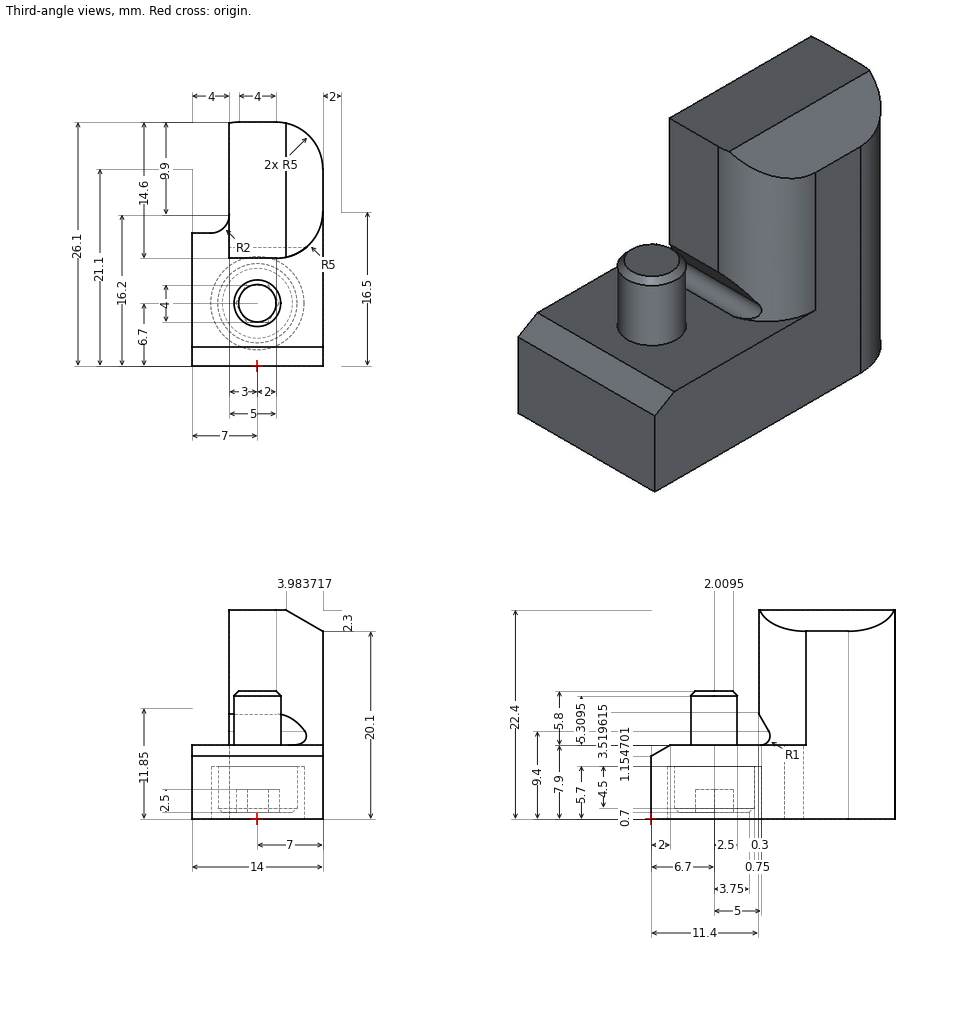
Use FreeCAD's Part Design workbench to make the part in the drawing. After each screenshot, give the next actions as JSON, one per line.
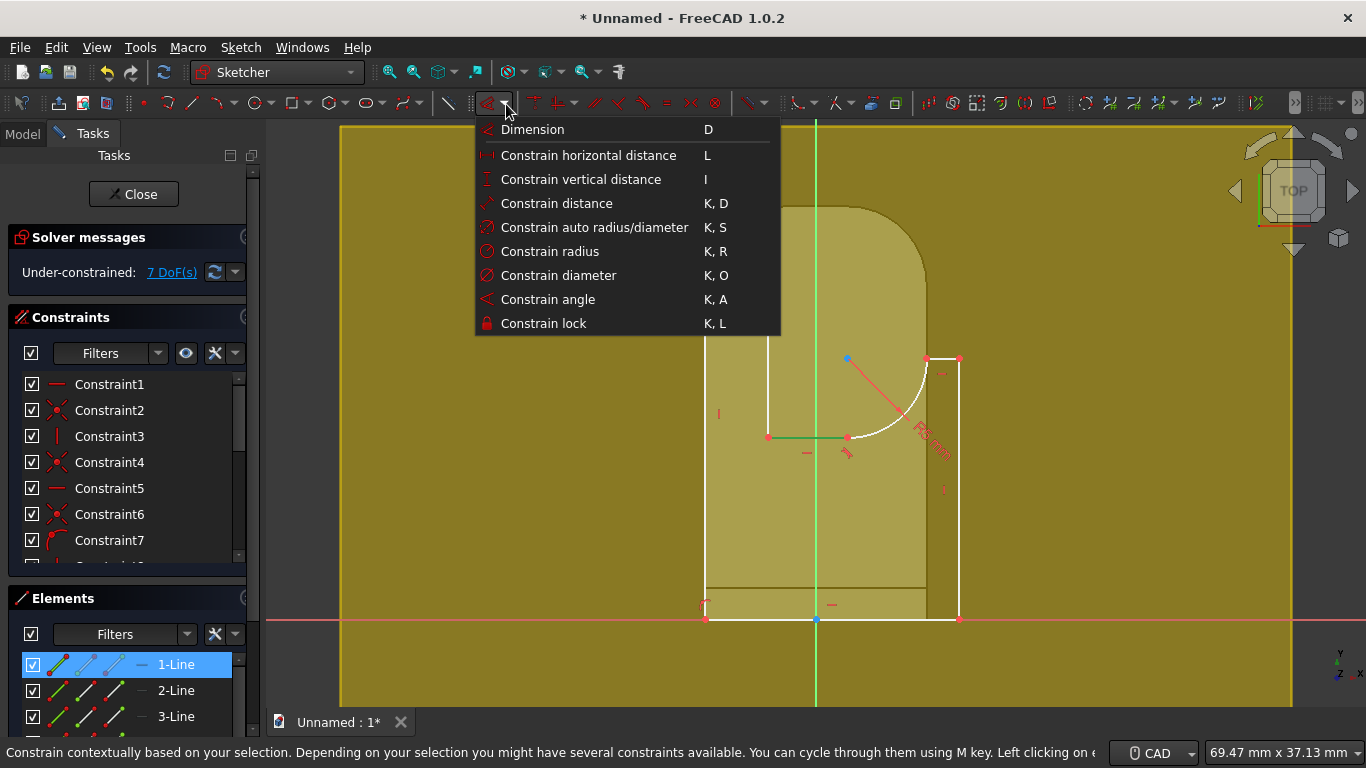
{"action": "left_click", "coordinate": [628, 155]}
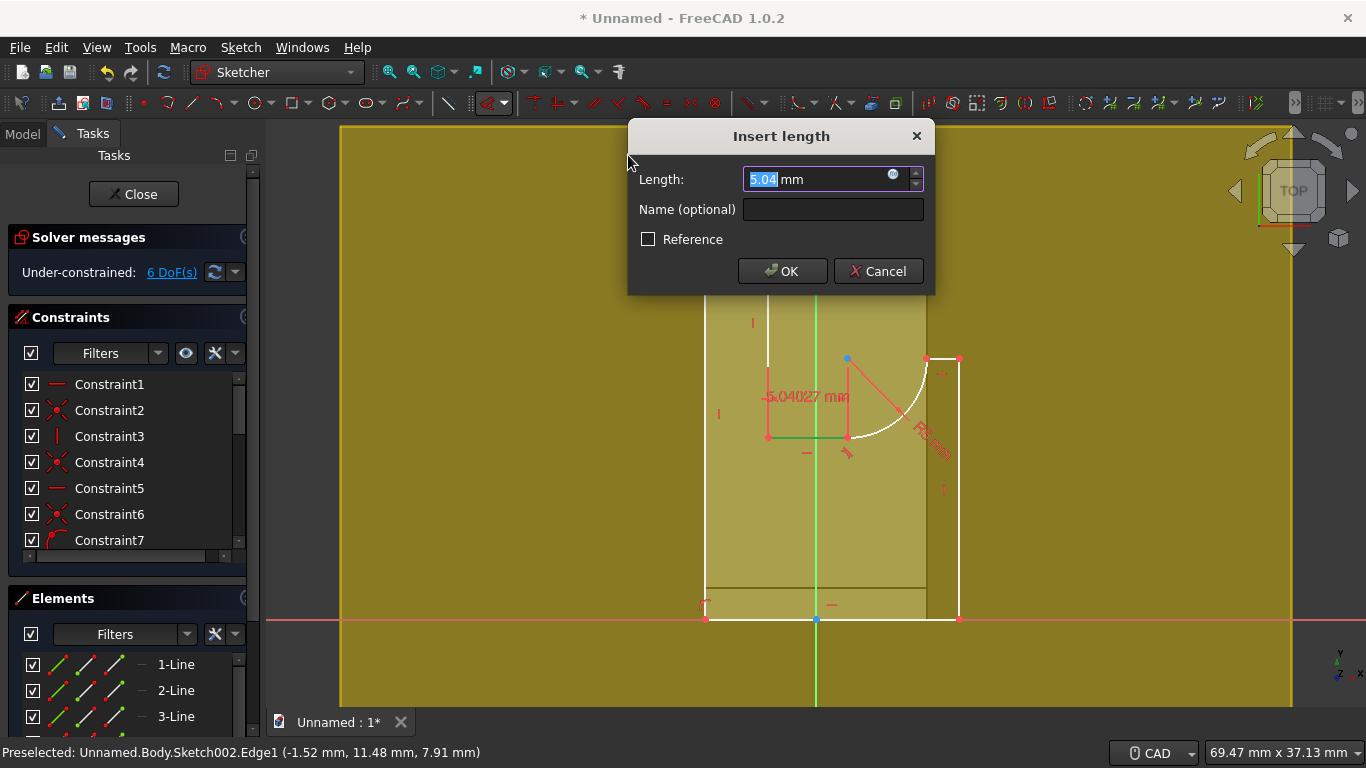
{"action": "type", "text": "5"}
{"action": "key", "text": "Return"}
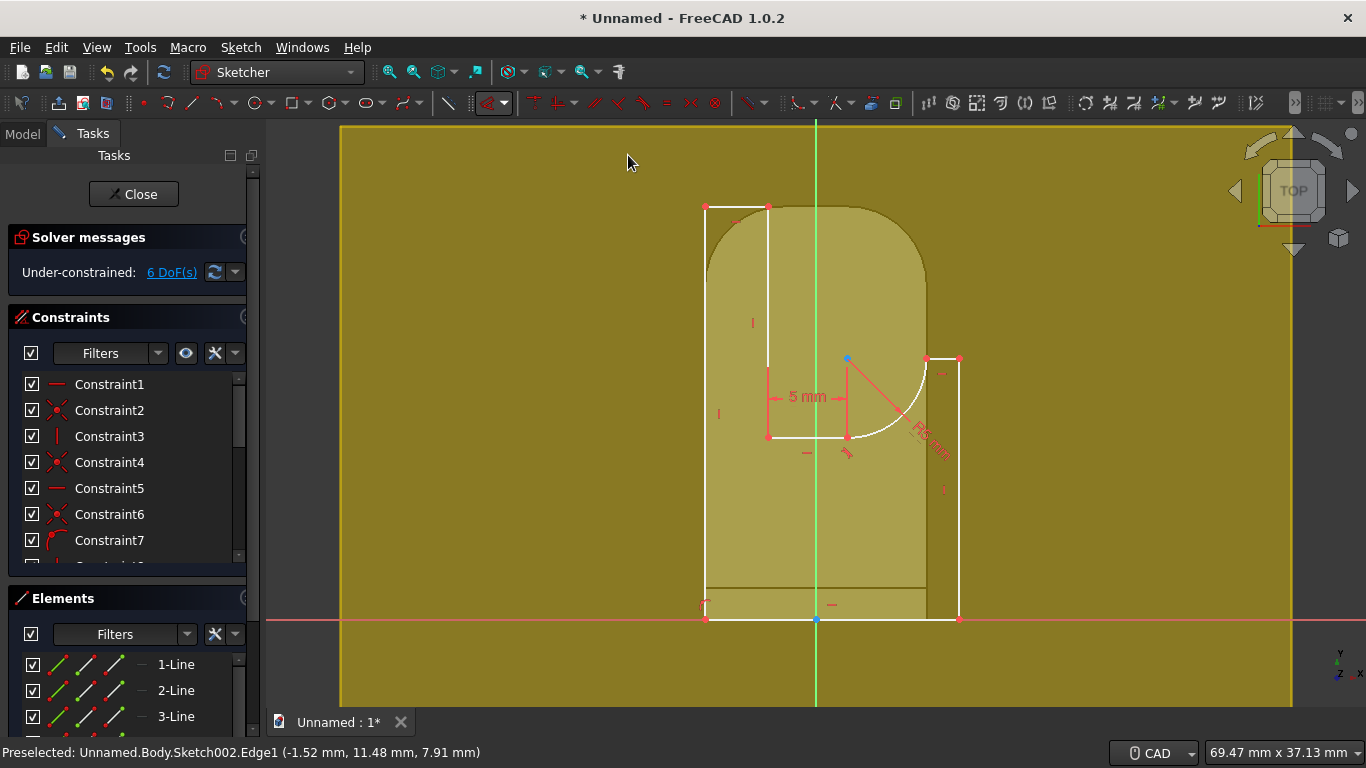
{"action": "left_click", "coordinate": [749, 207]}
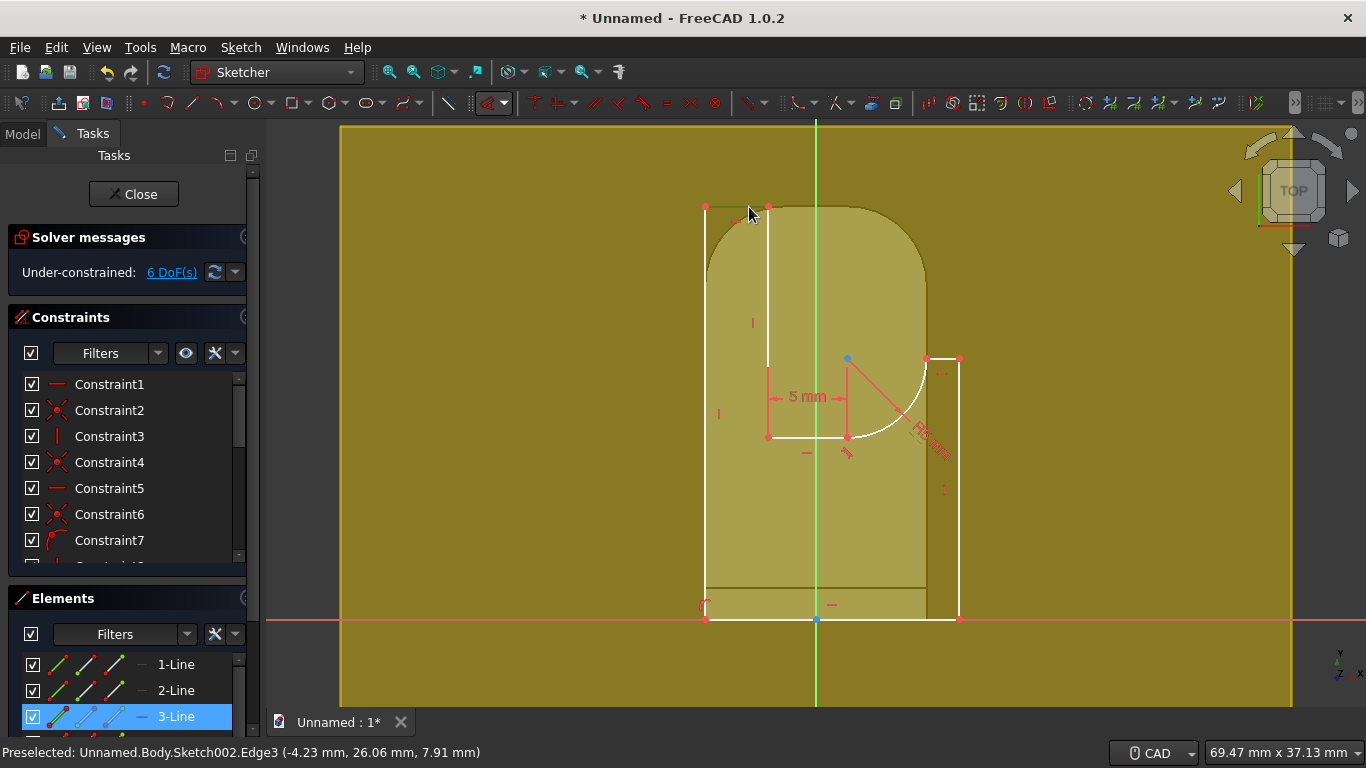
{"action": "key", "text": "l"}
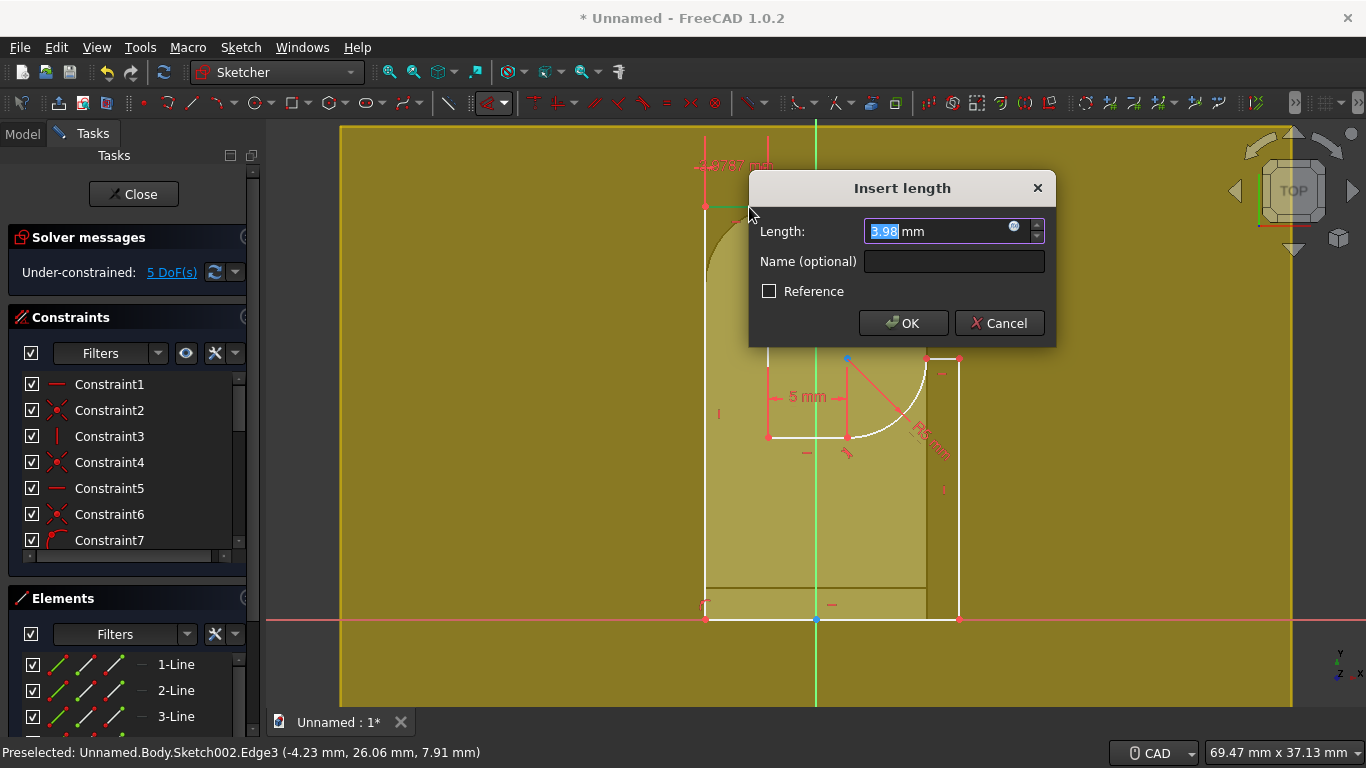
{"action": "type", "text": "4"}
{"action": "key", "text": "Return"}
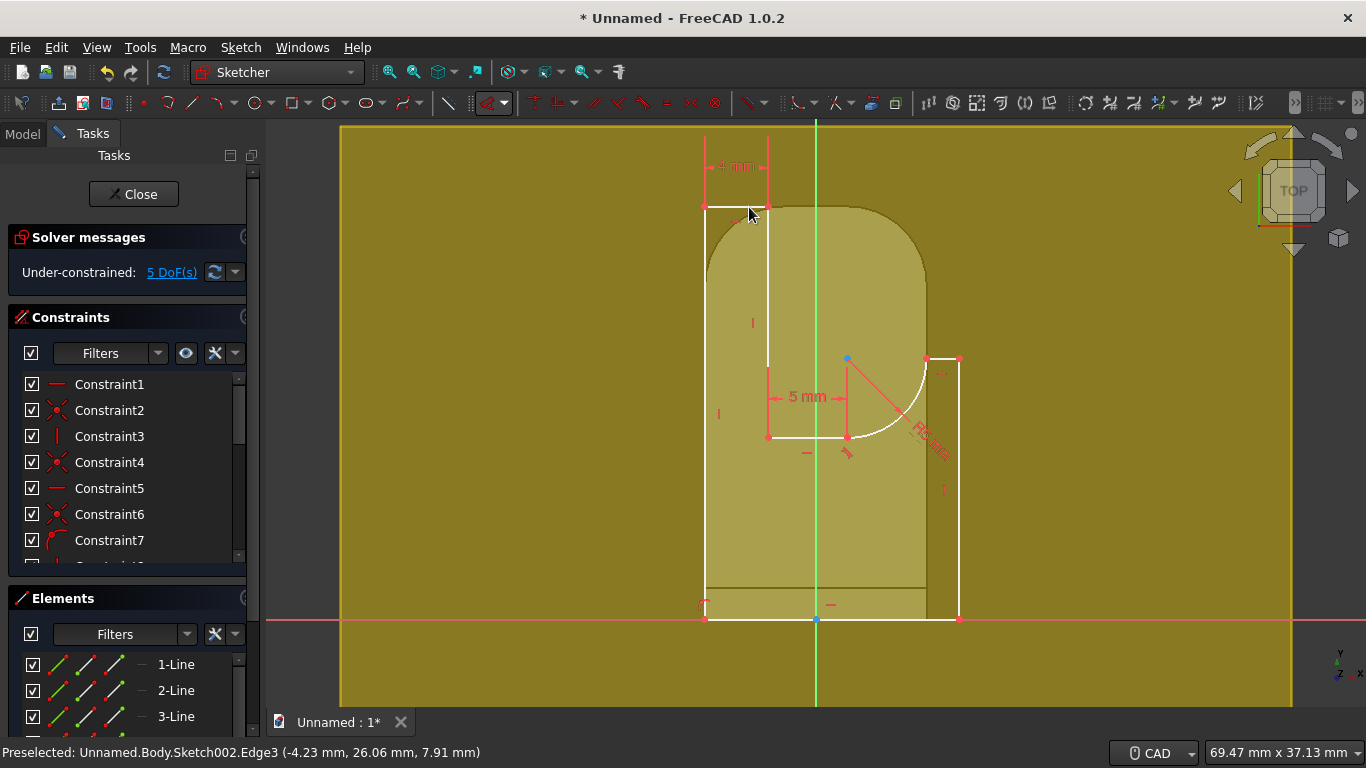
{"action": "scroll", "coordinate": [949, 359], "scroll_direction": "up", "scroll_amount": 2}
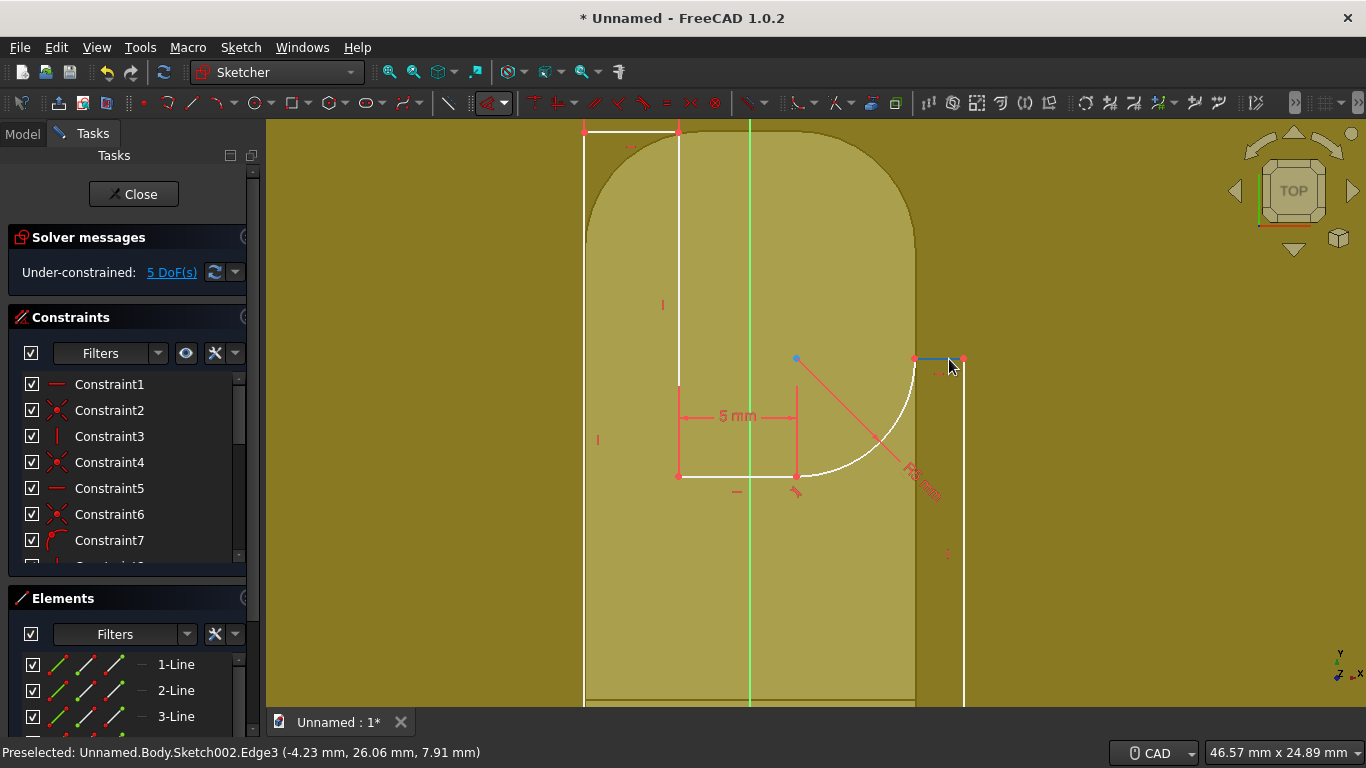
{"action": "left_click", "coordinate": [949, 359]}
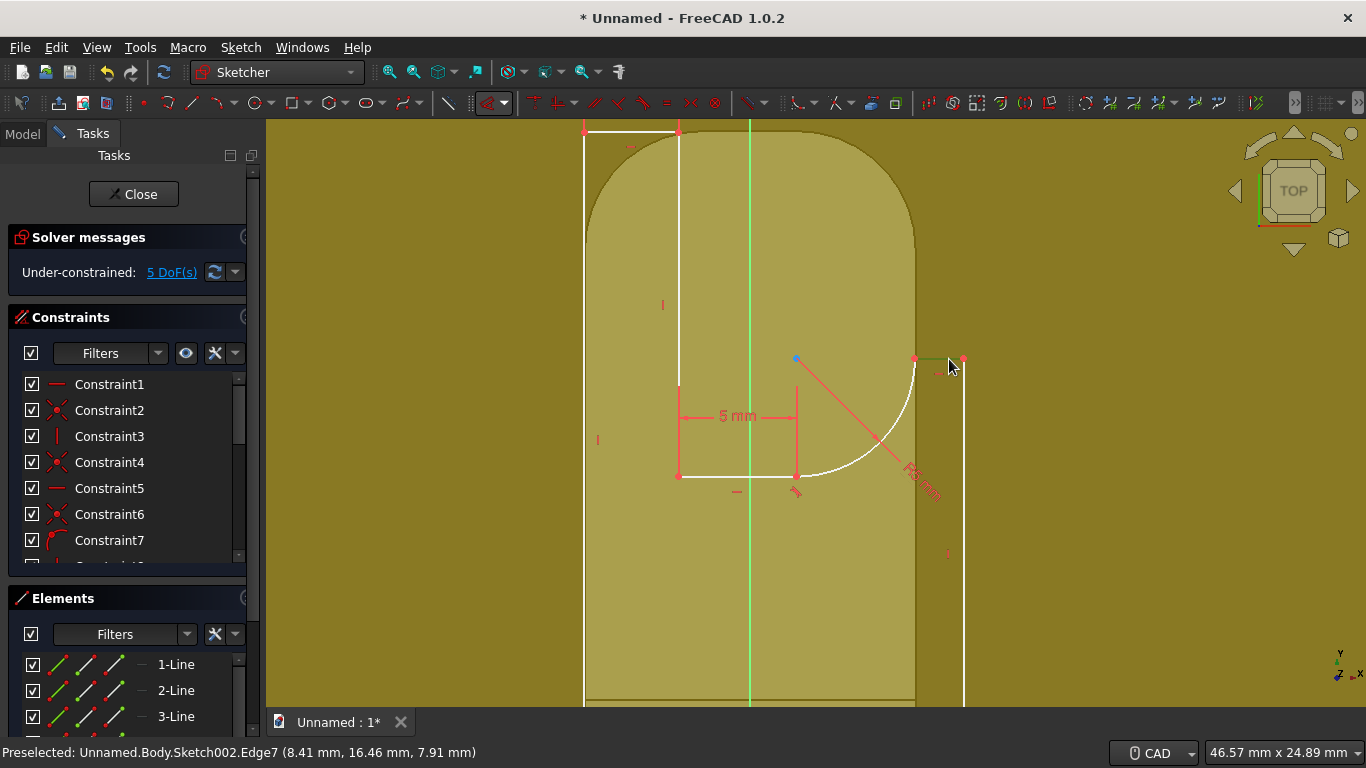
{"action": "left_click", "coordinate": [506, 104]}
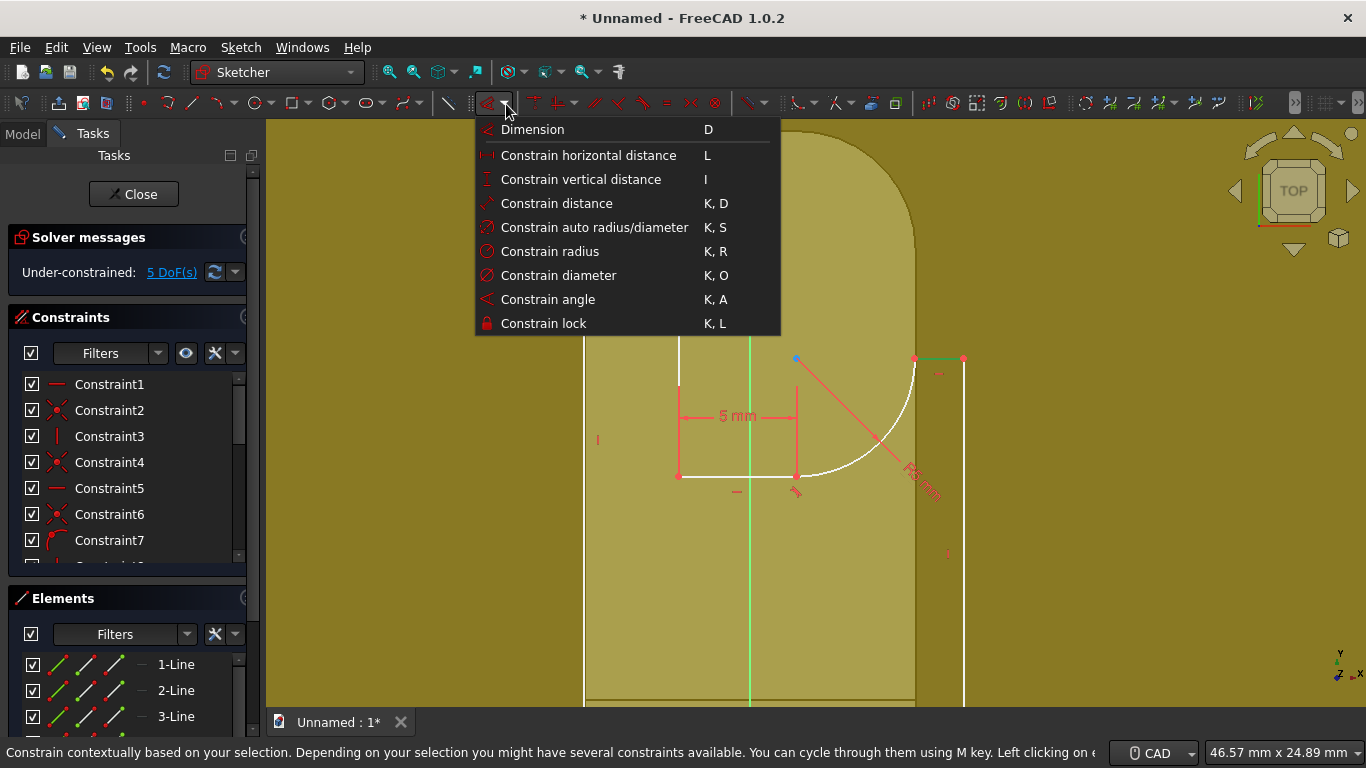
{"action": "left_click", "coordinate": [628, 155]}